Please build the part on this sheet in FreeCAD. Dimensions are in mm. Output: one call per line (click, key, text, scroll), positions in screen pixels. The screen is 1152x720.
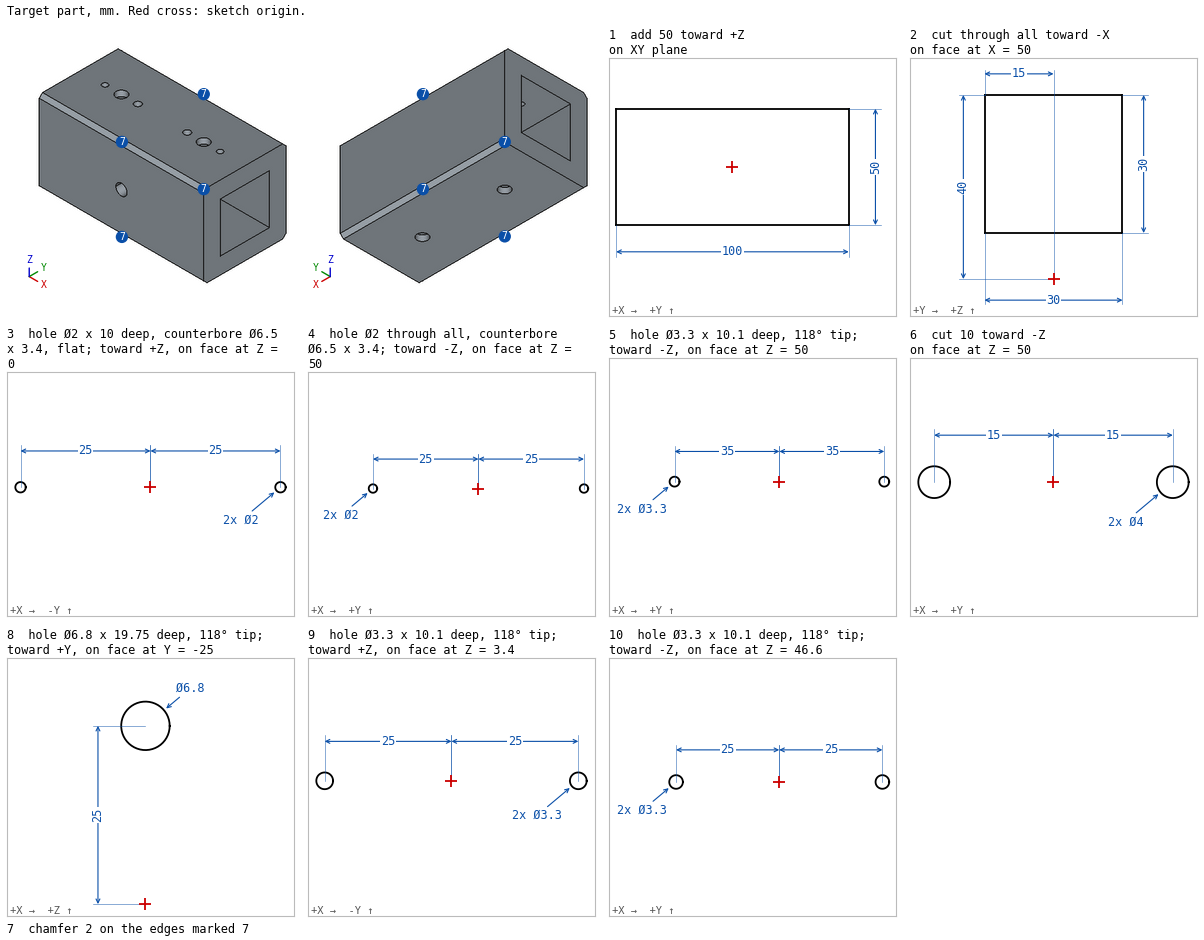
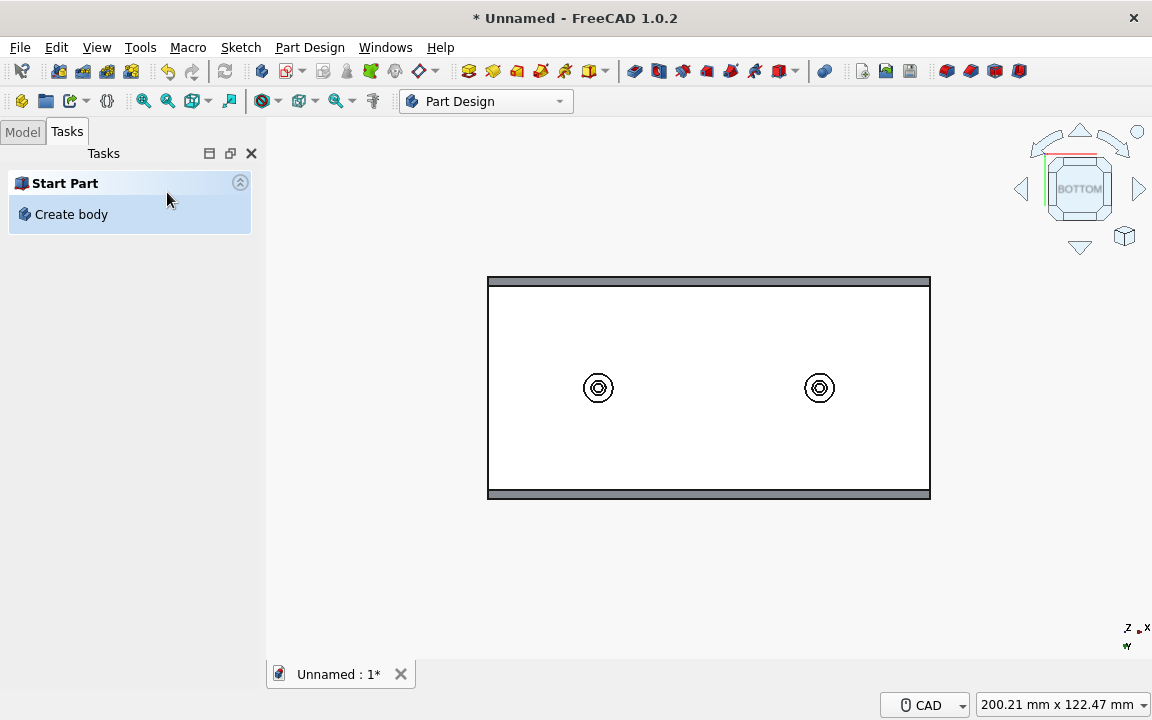
key(0)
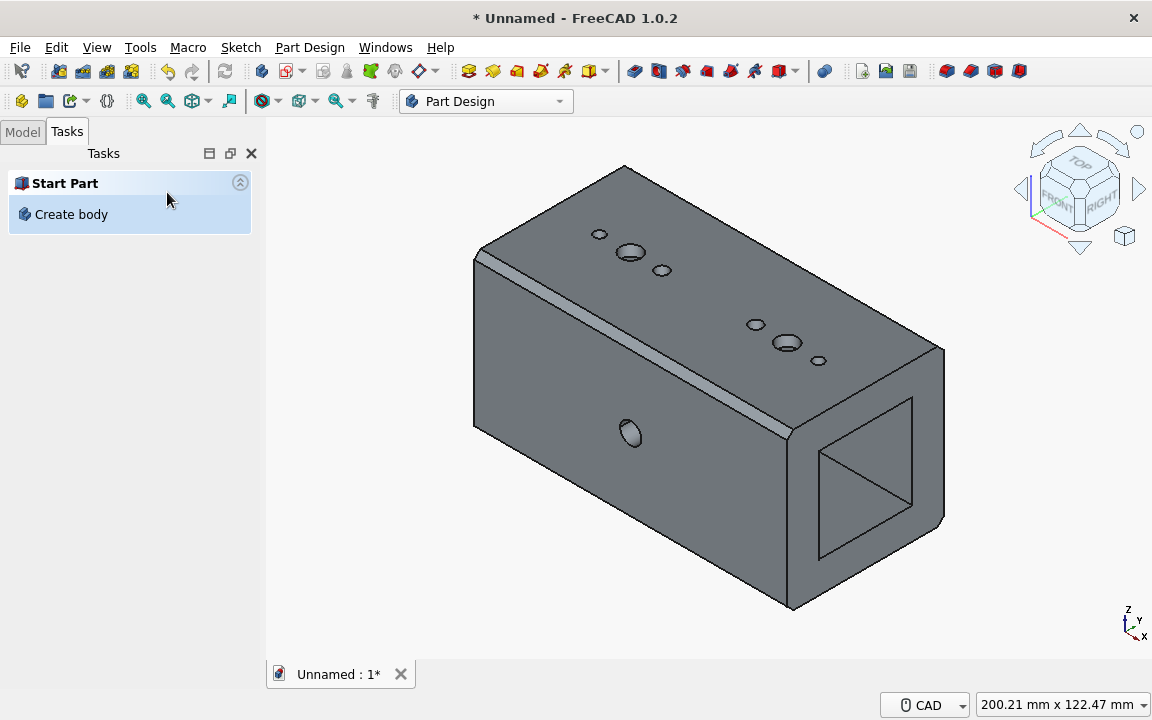
scroll(784, 359, up, 5)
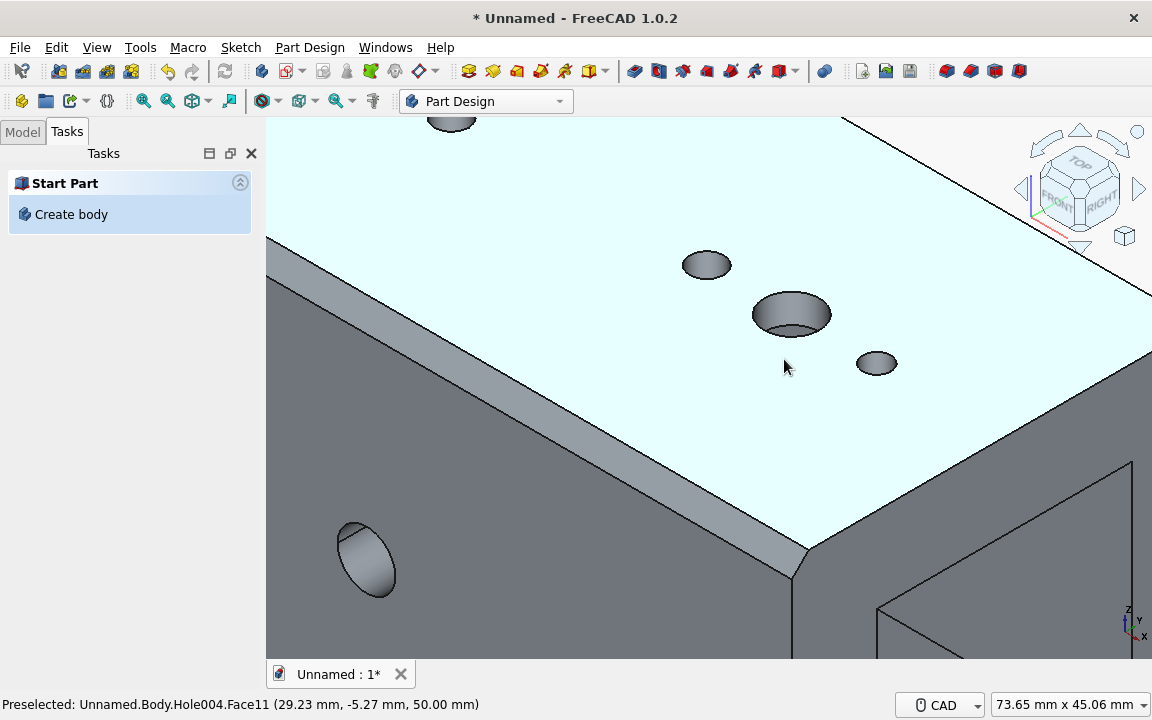
click(144, 102)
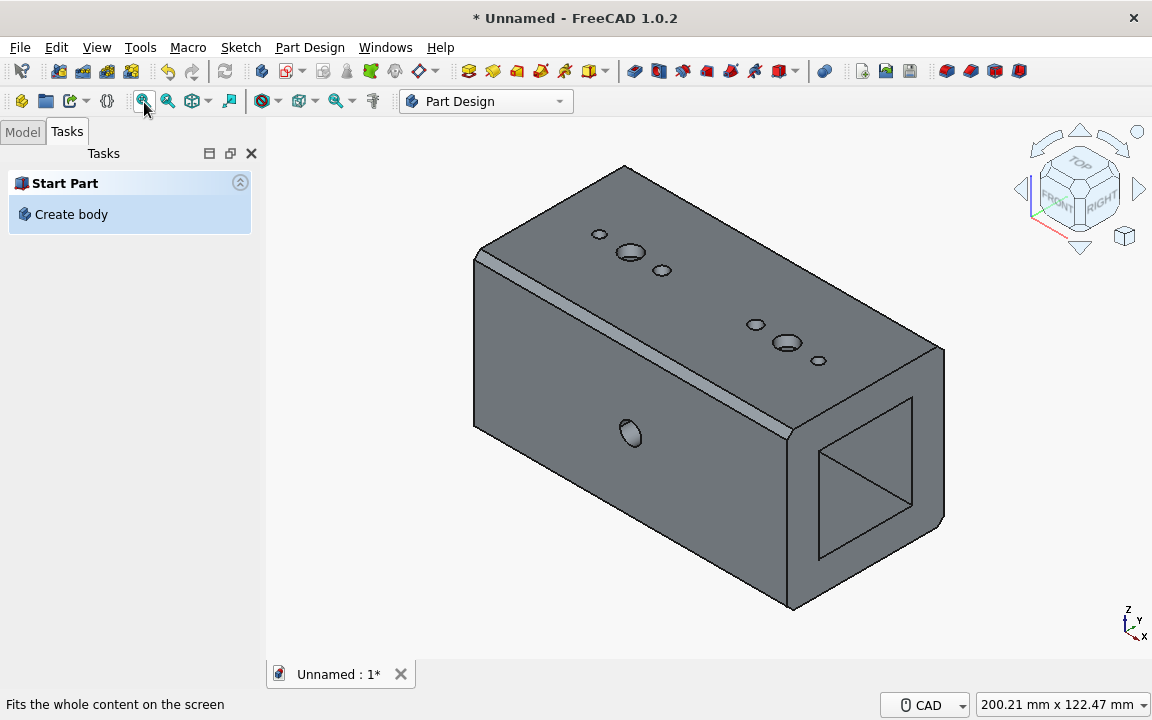
key(2)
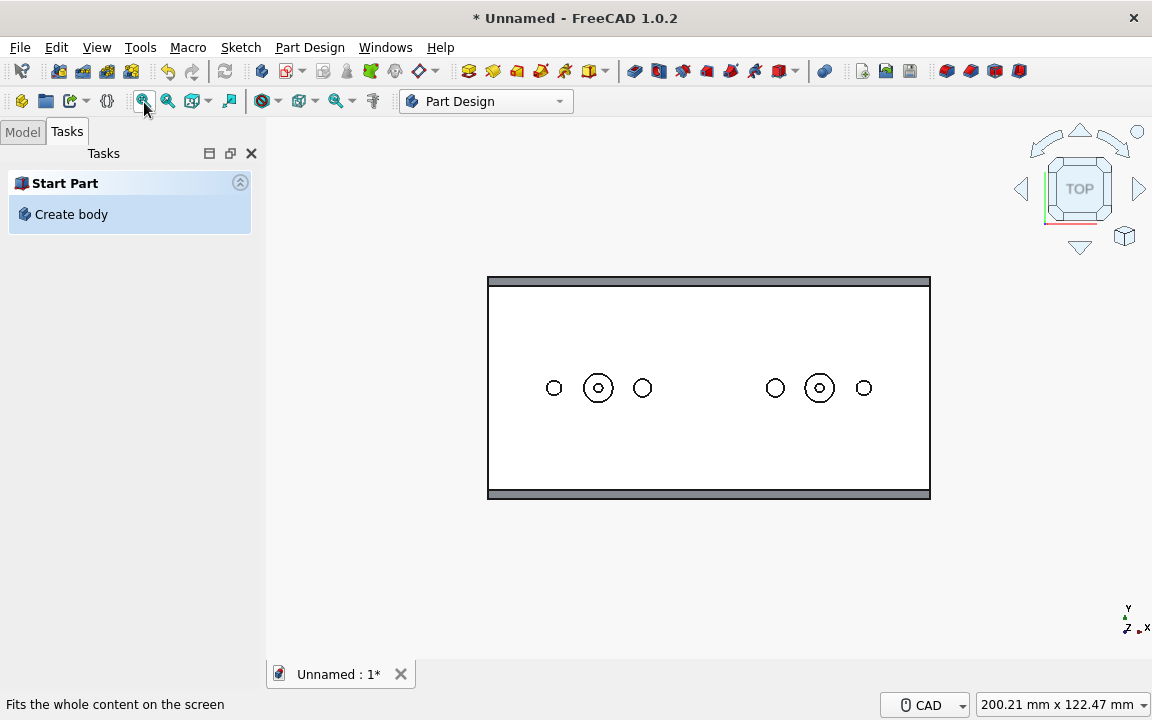
scroll(824, 395, up, 5)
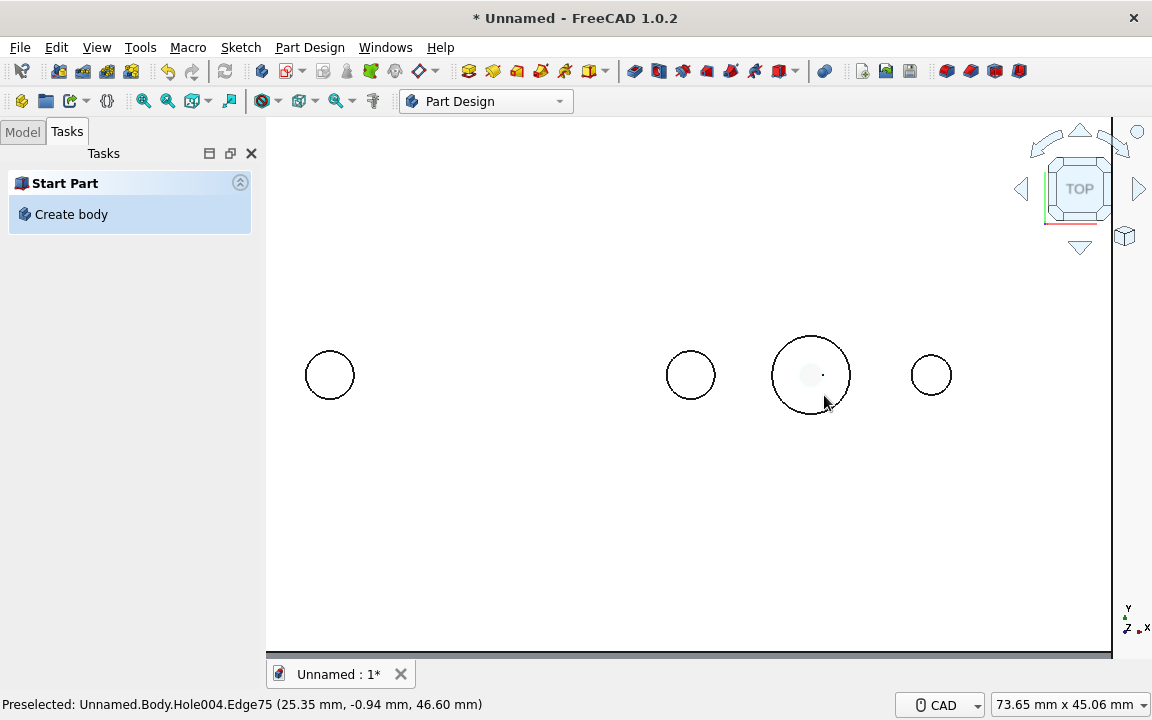
click(822, 396)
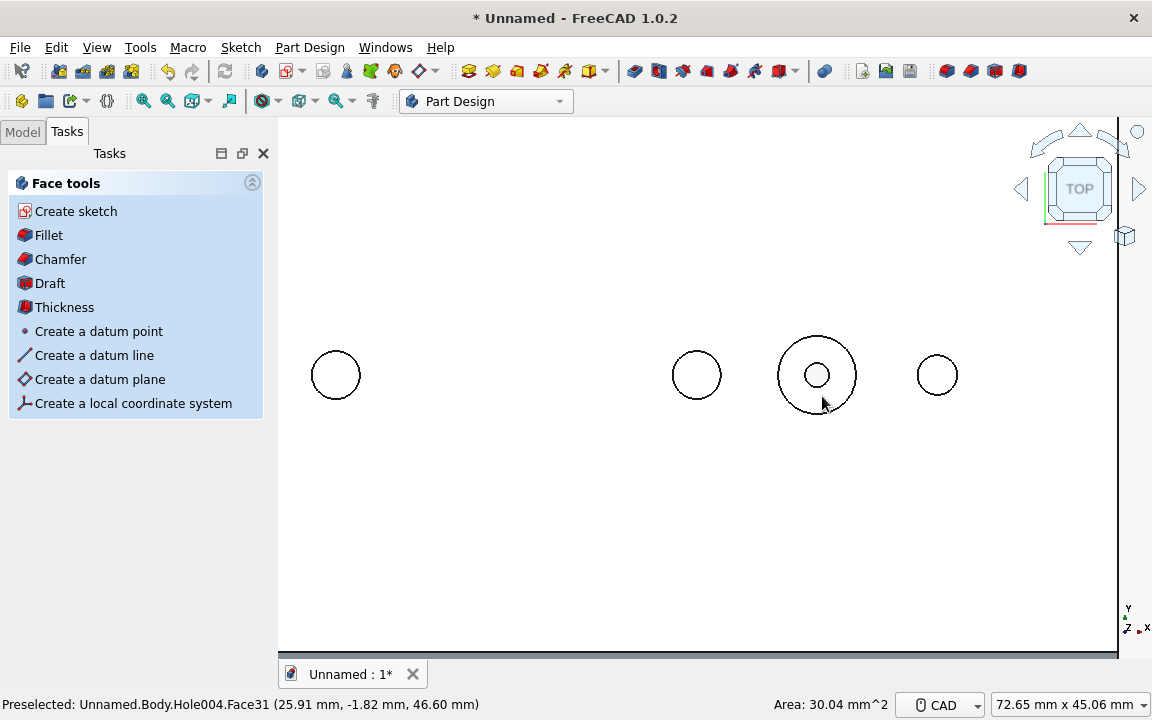
click(286, 72)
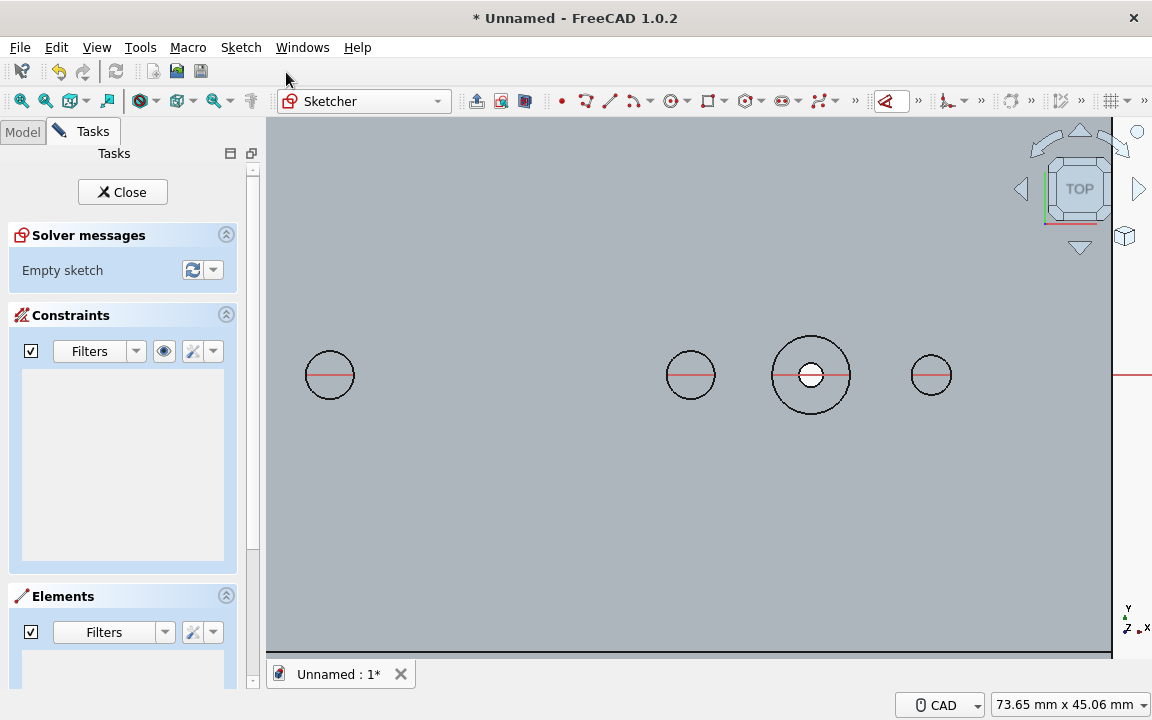
key(q)
key(s)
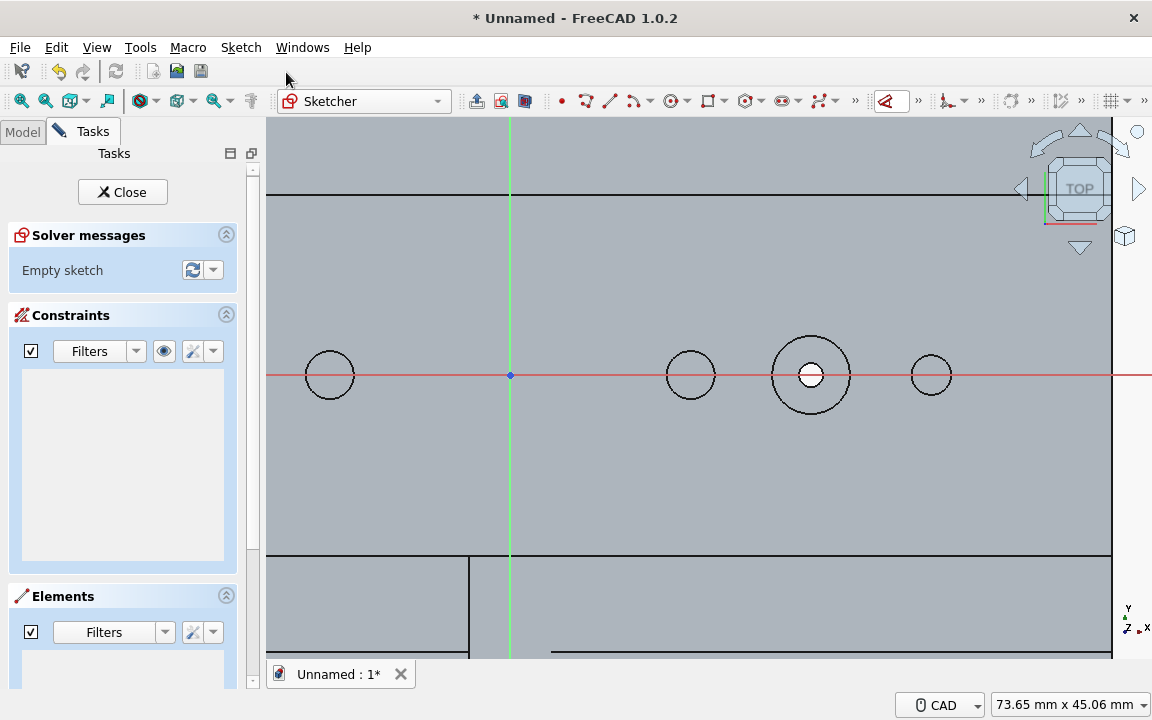
scroll(987, 446, down, 1)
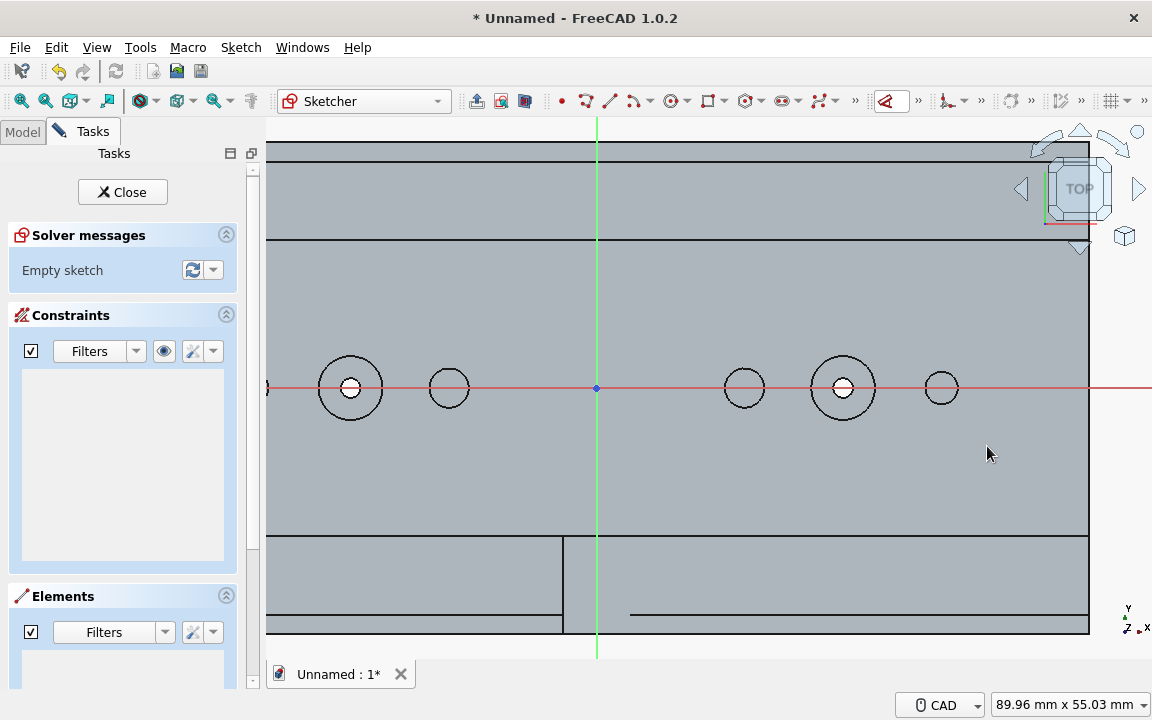
click(672, 102)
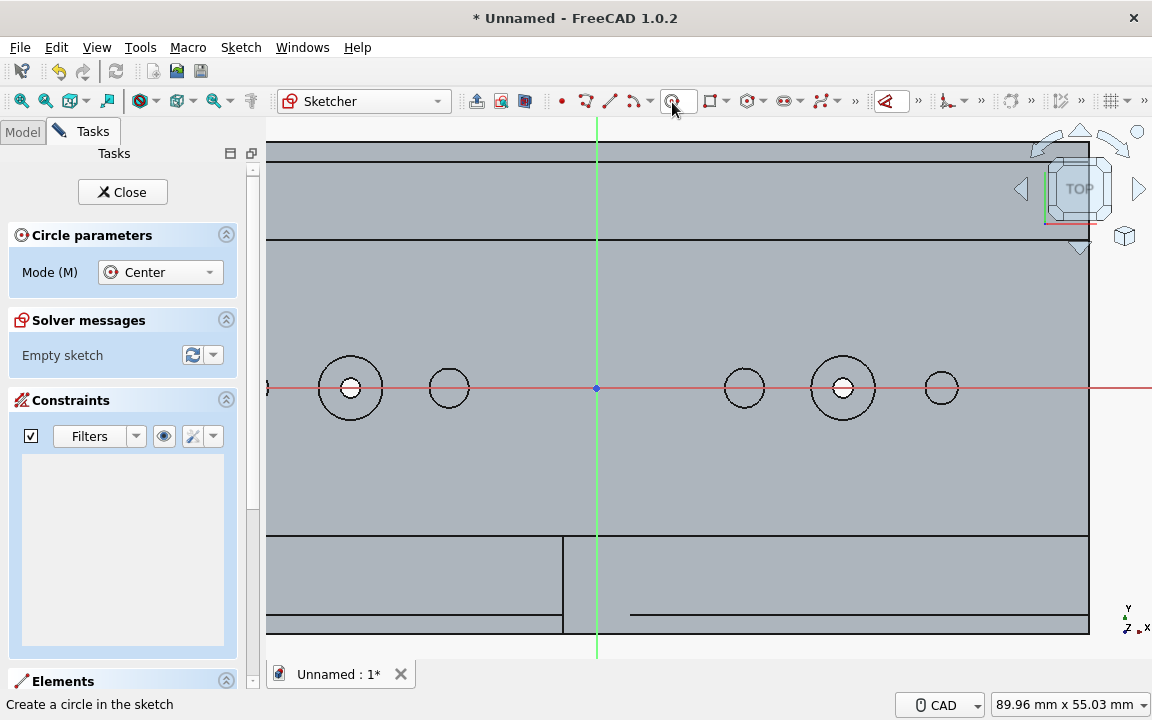
scroll(351, 388, up, 2)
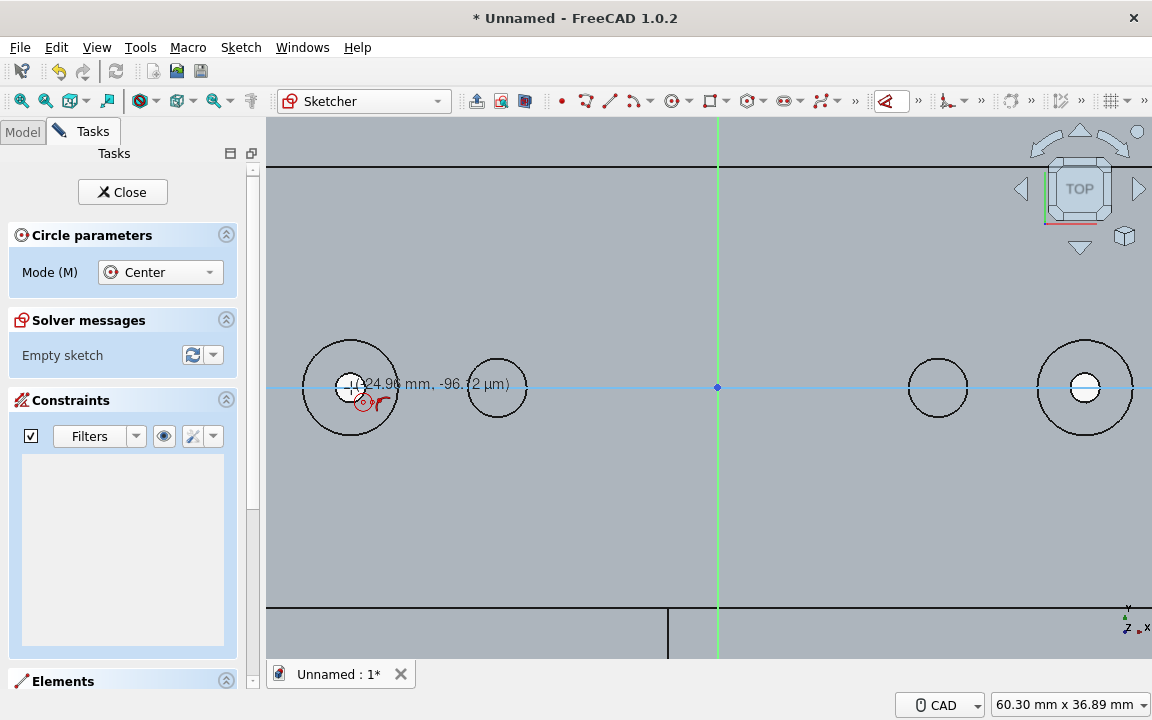
click(350, 388)
move(368, 371)